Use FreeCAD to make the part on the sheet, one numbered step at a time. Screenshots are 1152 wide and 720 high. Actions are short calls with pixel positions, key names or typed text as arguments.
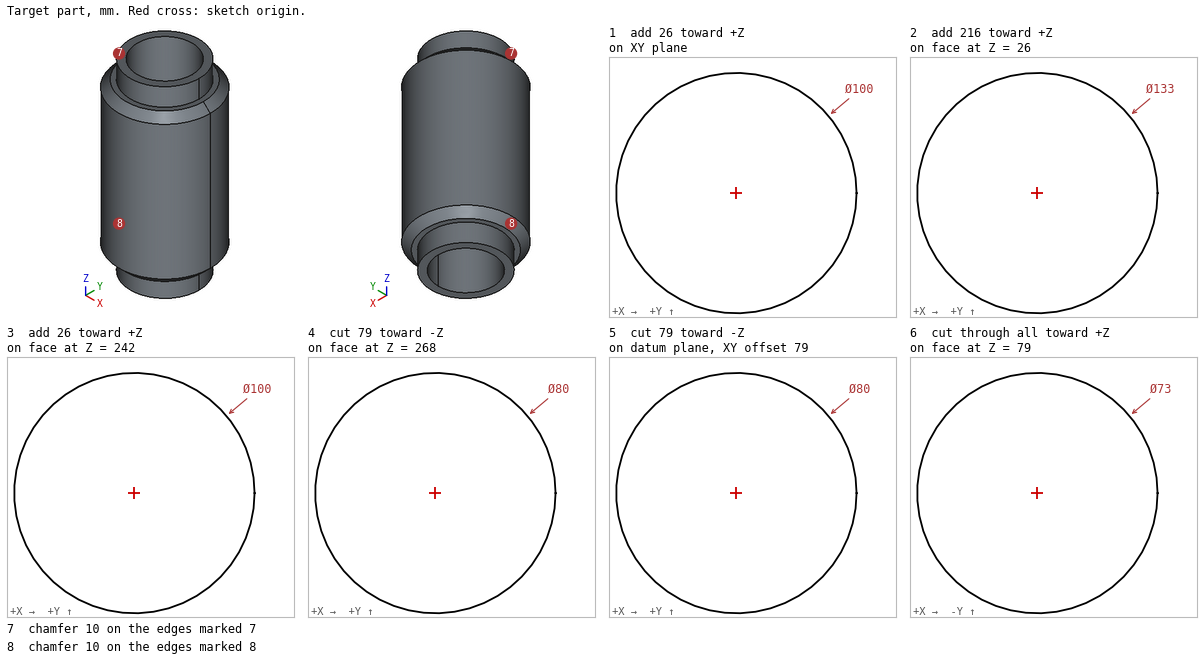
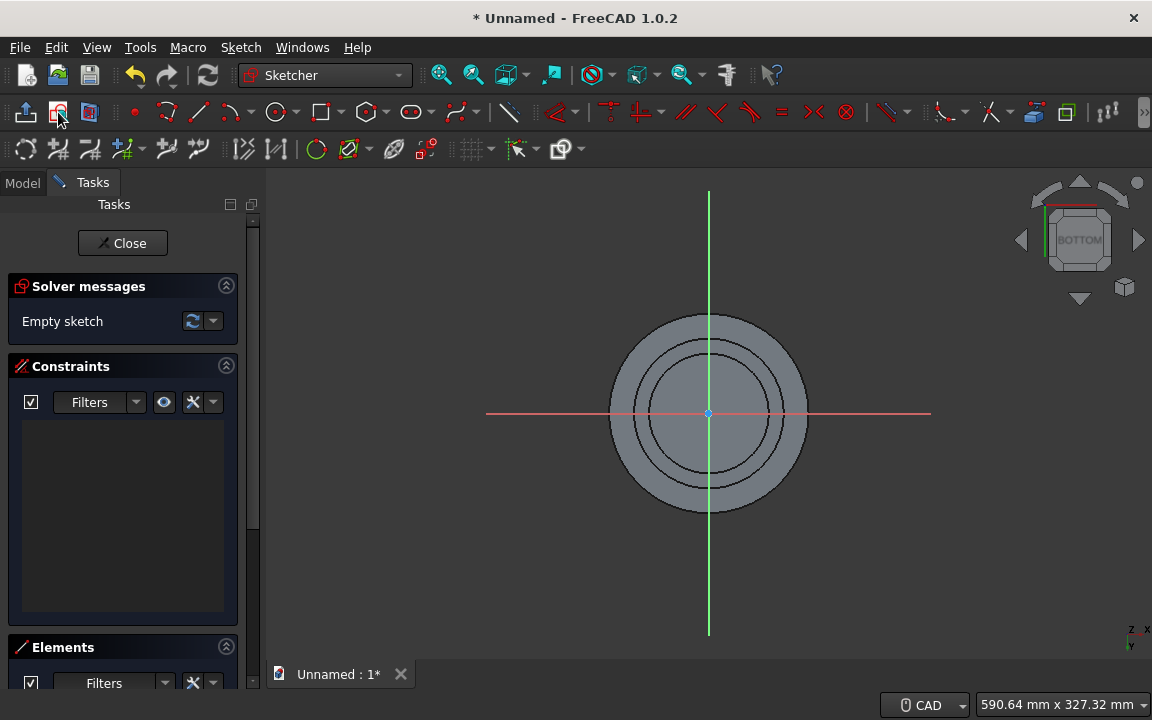
scroll(749, 414, up, 5)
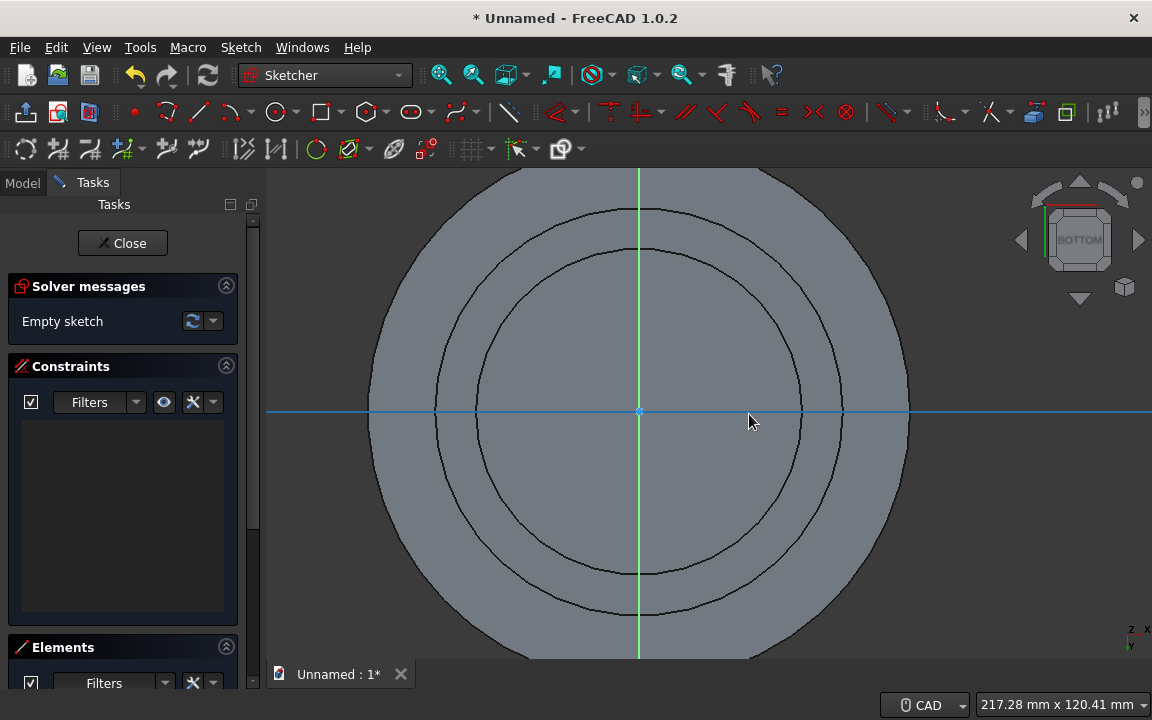
key(g)
key(c)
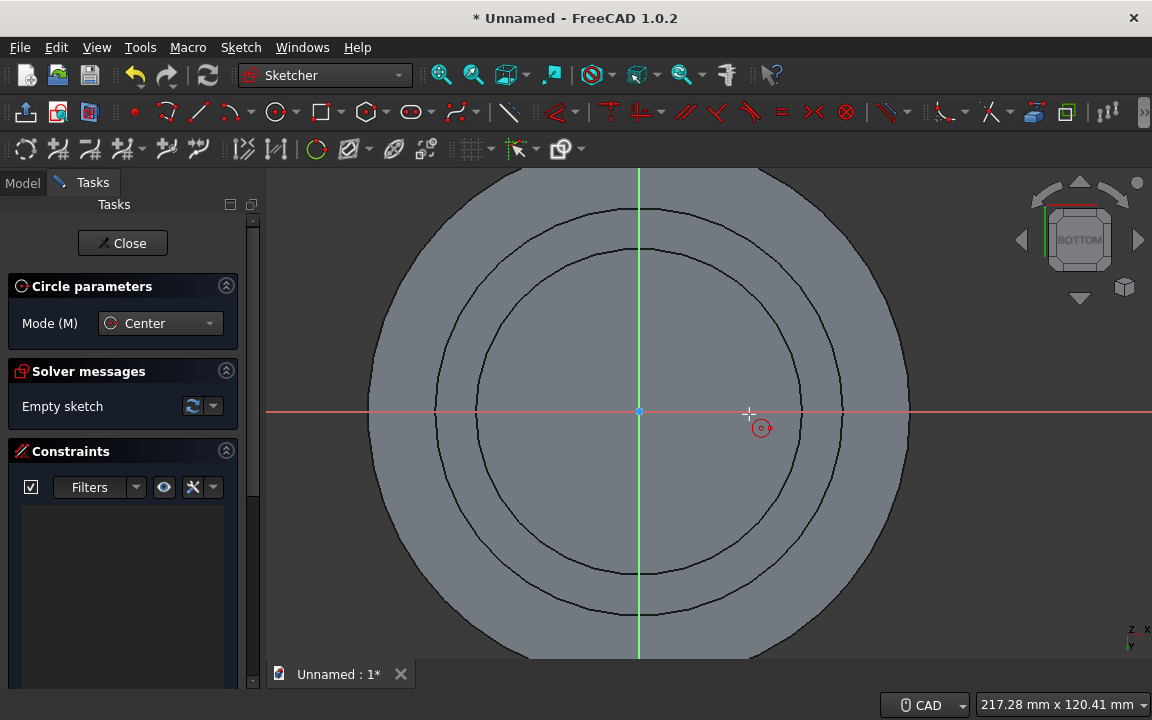
click(639, 412)
move(744, 307)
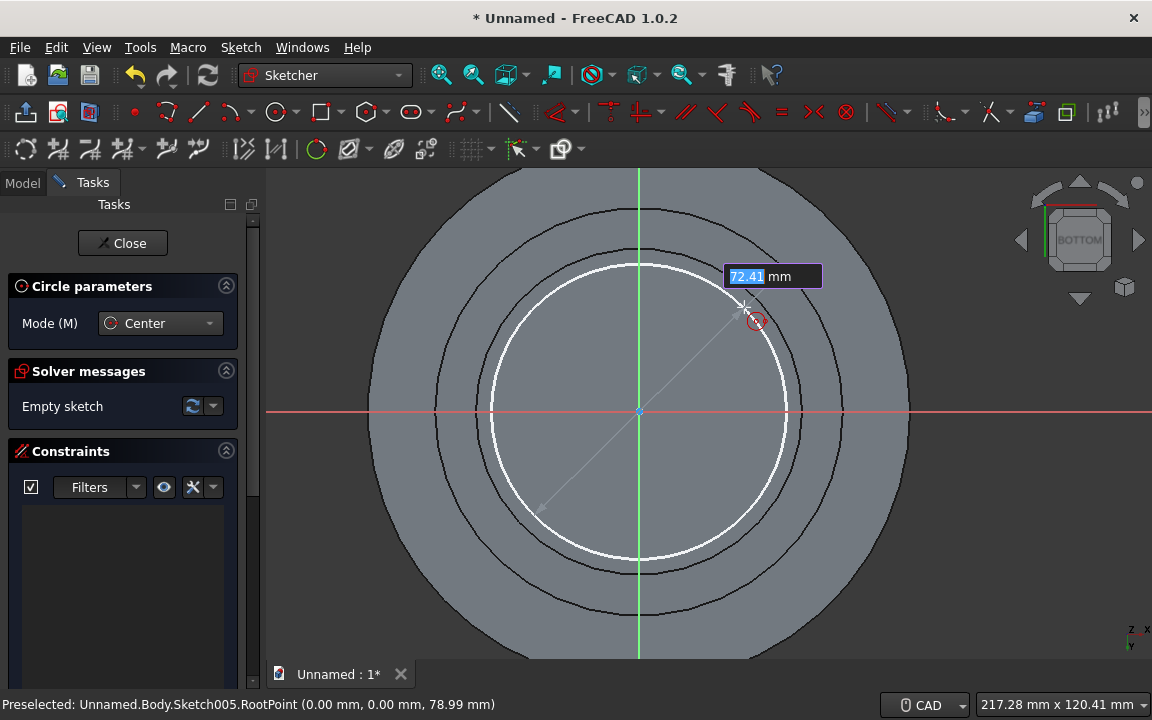
text(73)
key(Return)
key(Escape)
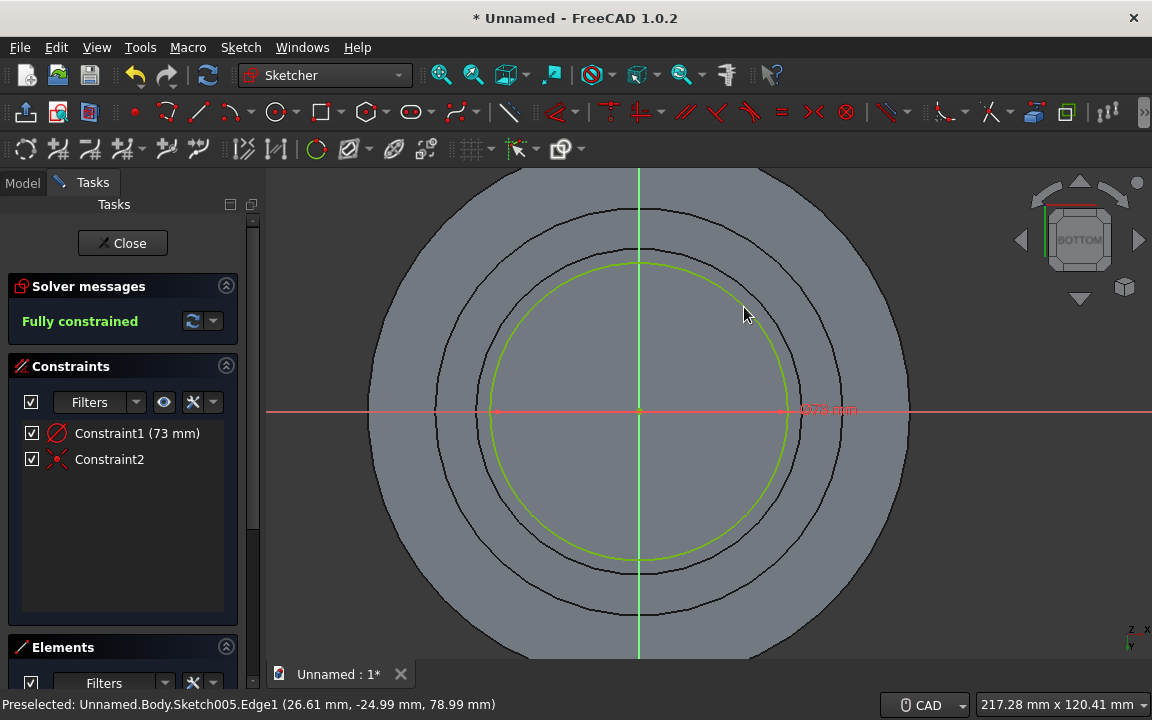
click(123, 243)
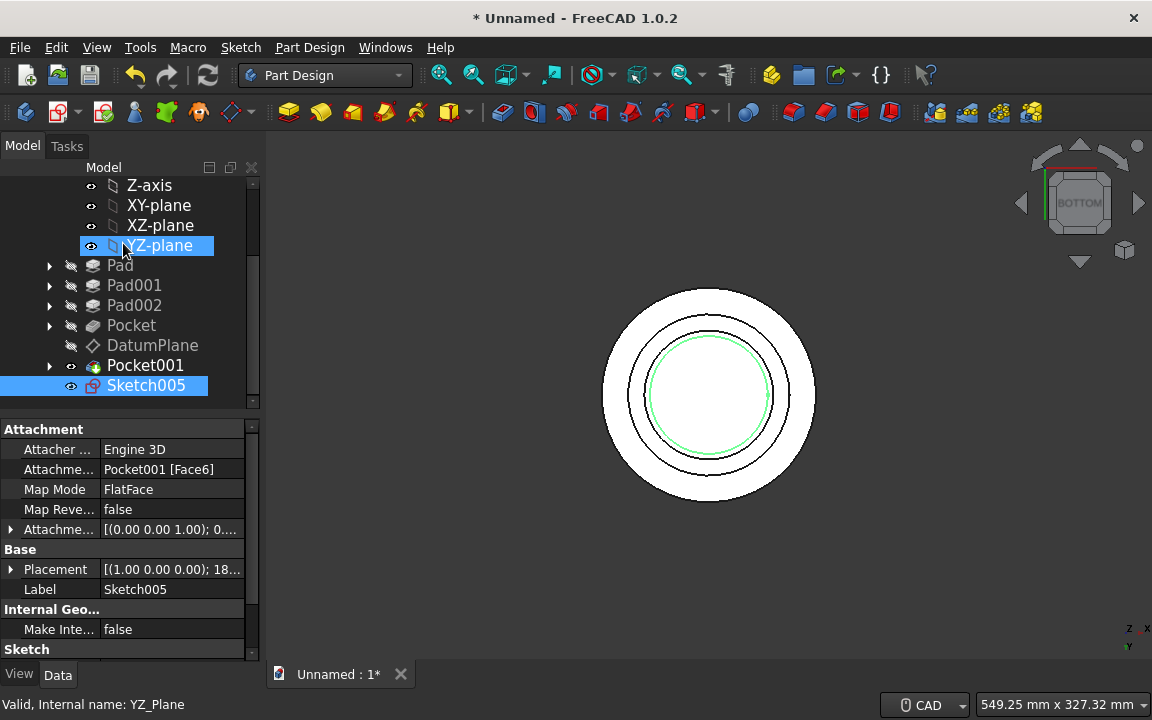
click(504, 112)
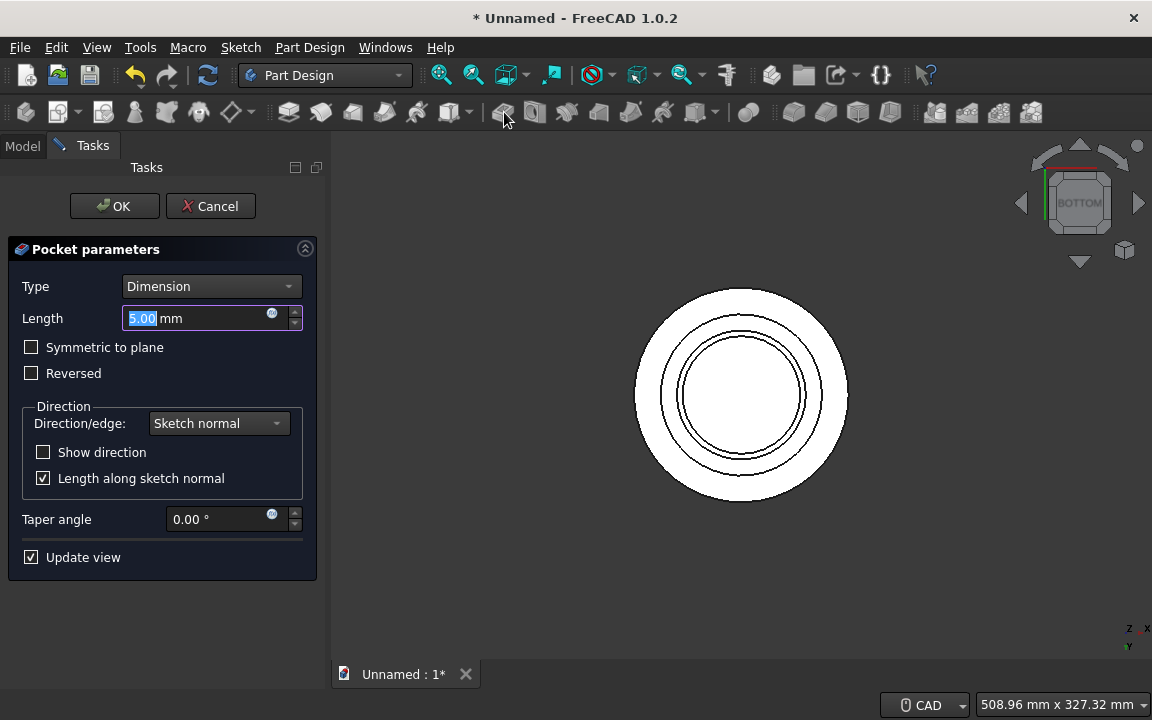
click(212, 286)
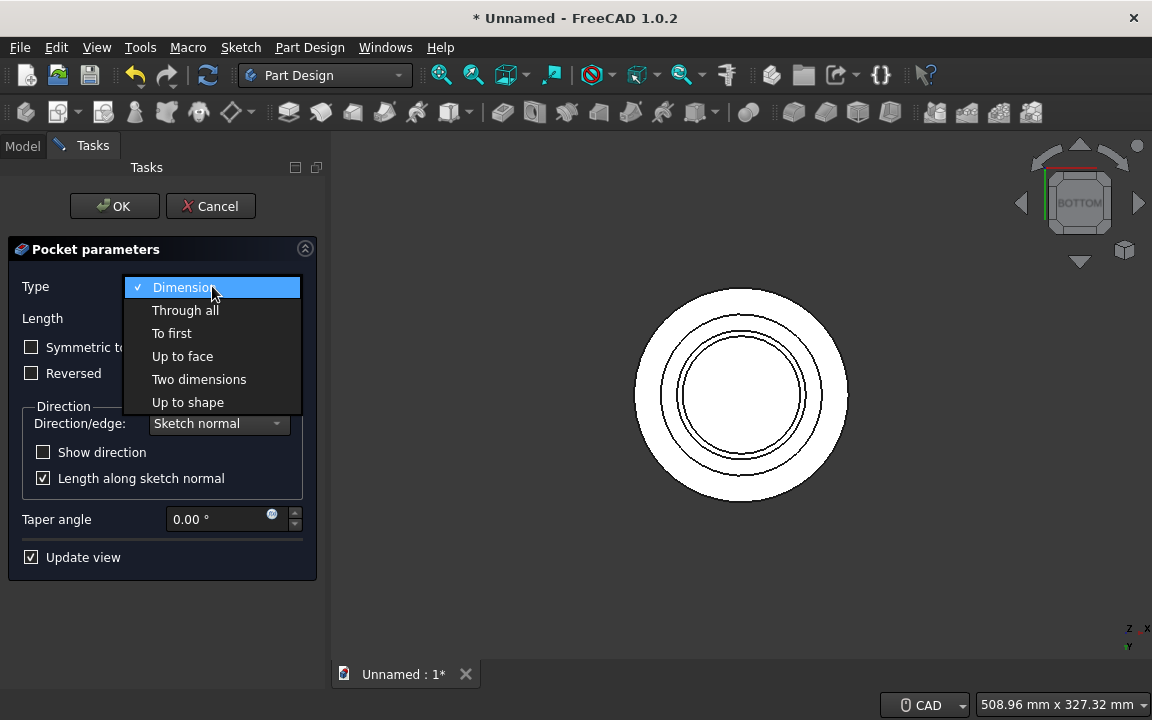
click(212, 310)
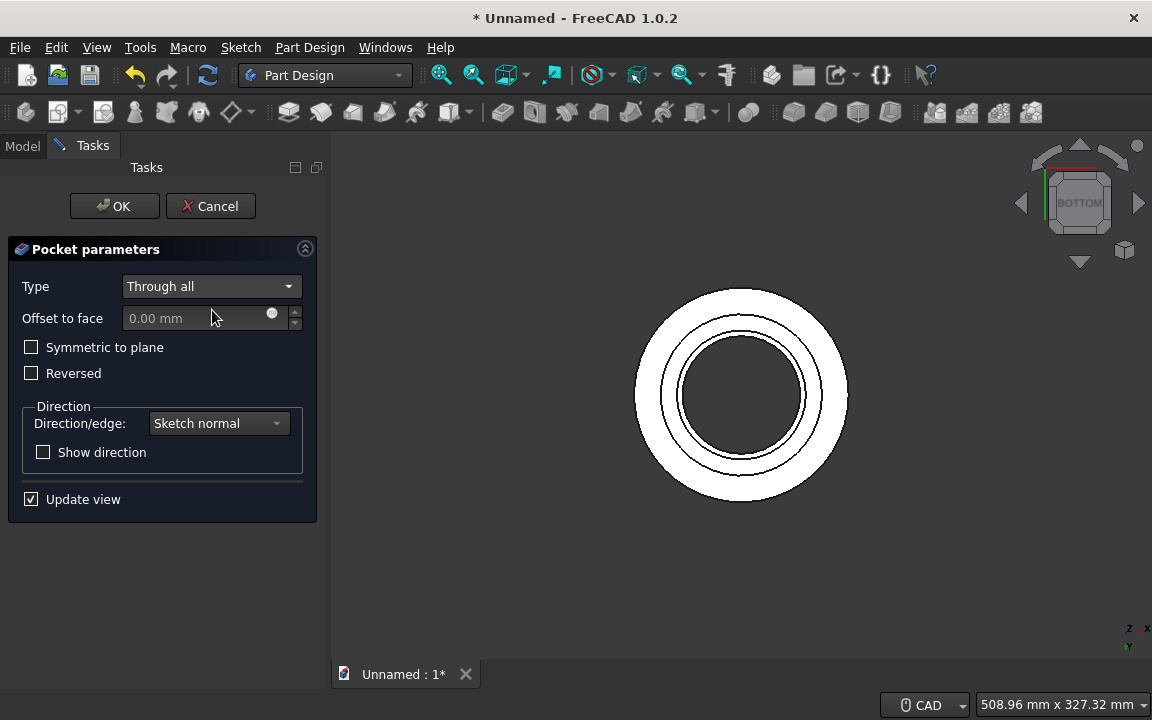
click(115, 206)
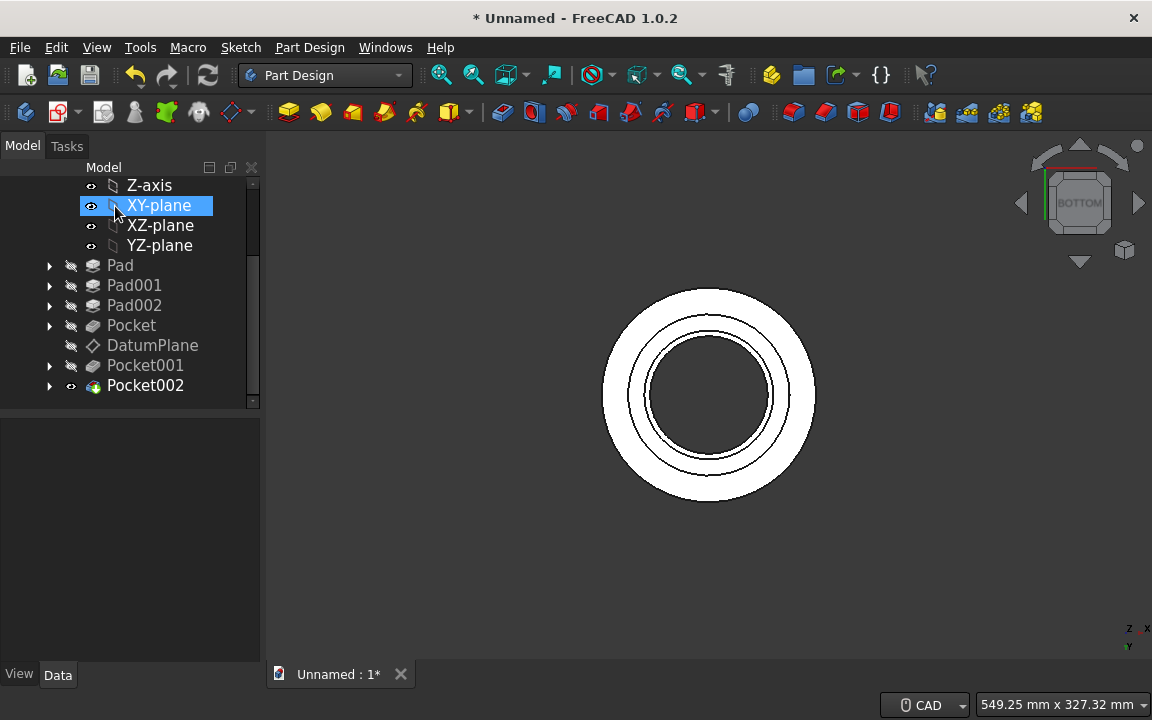
key(v)
key(f)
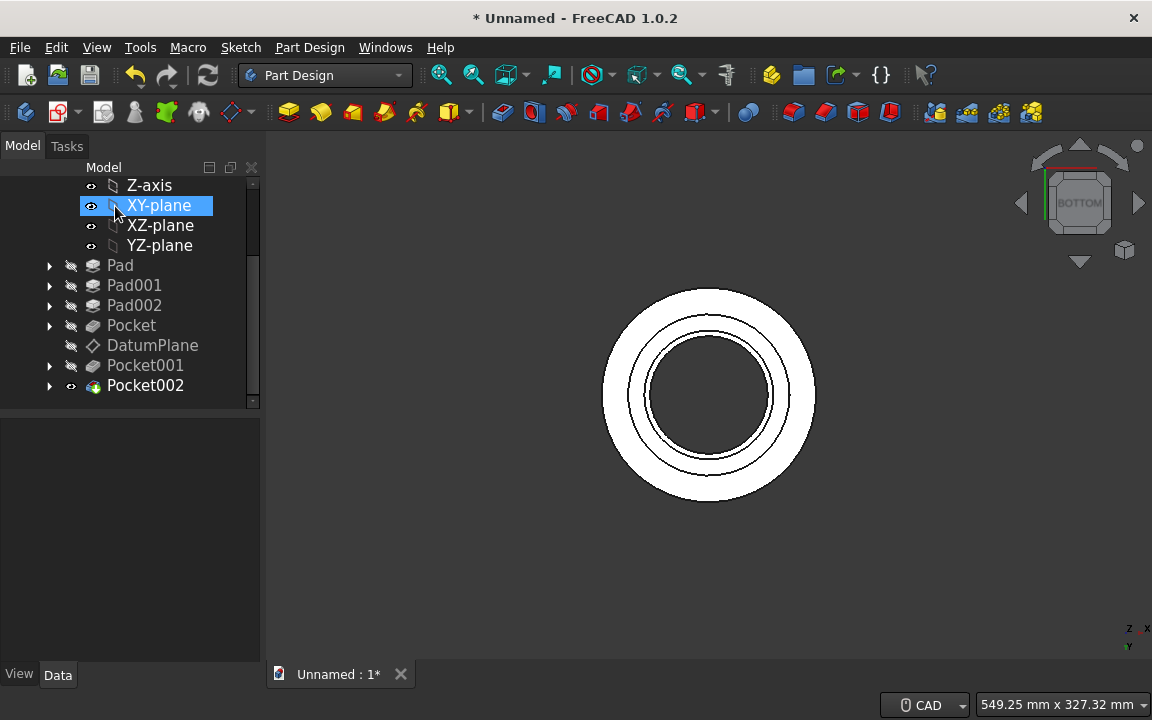
key(0)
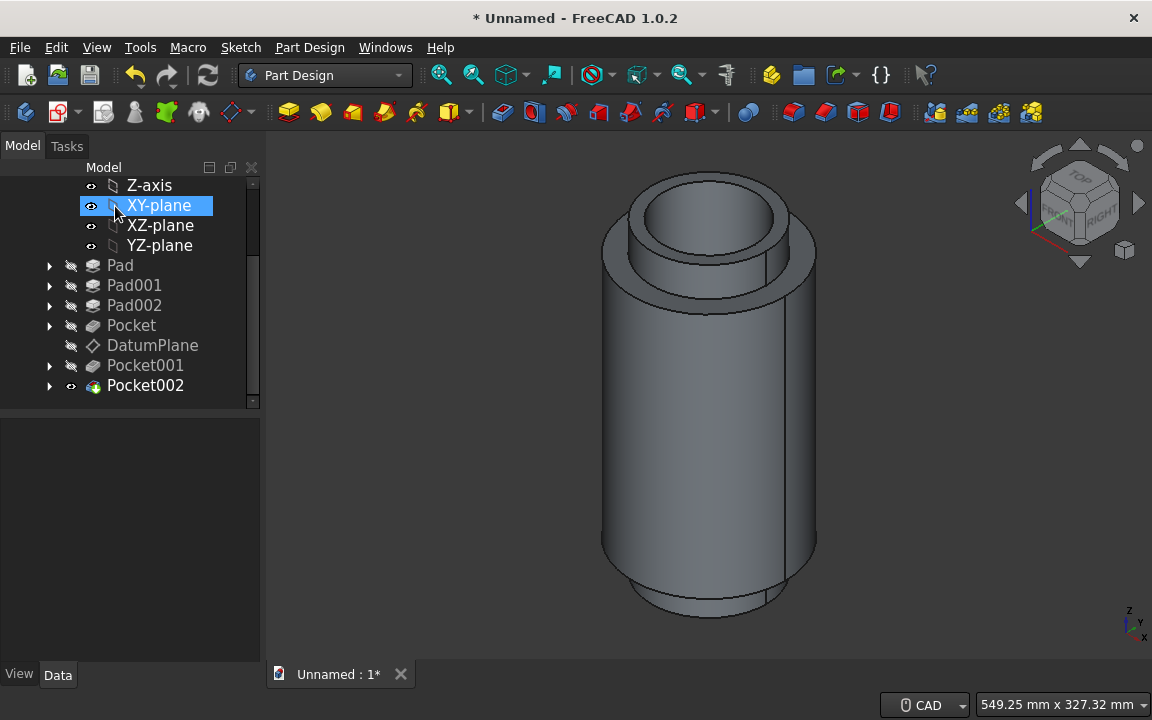
key(v)
key(f)